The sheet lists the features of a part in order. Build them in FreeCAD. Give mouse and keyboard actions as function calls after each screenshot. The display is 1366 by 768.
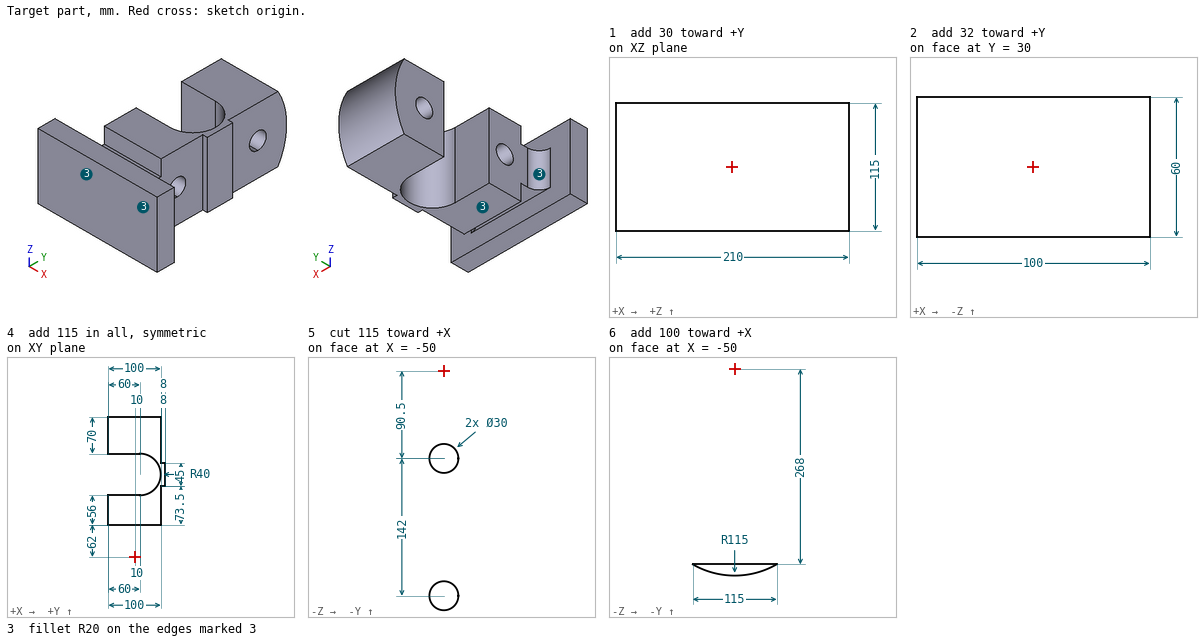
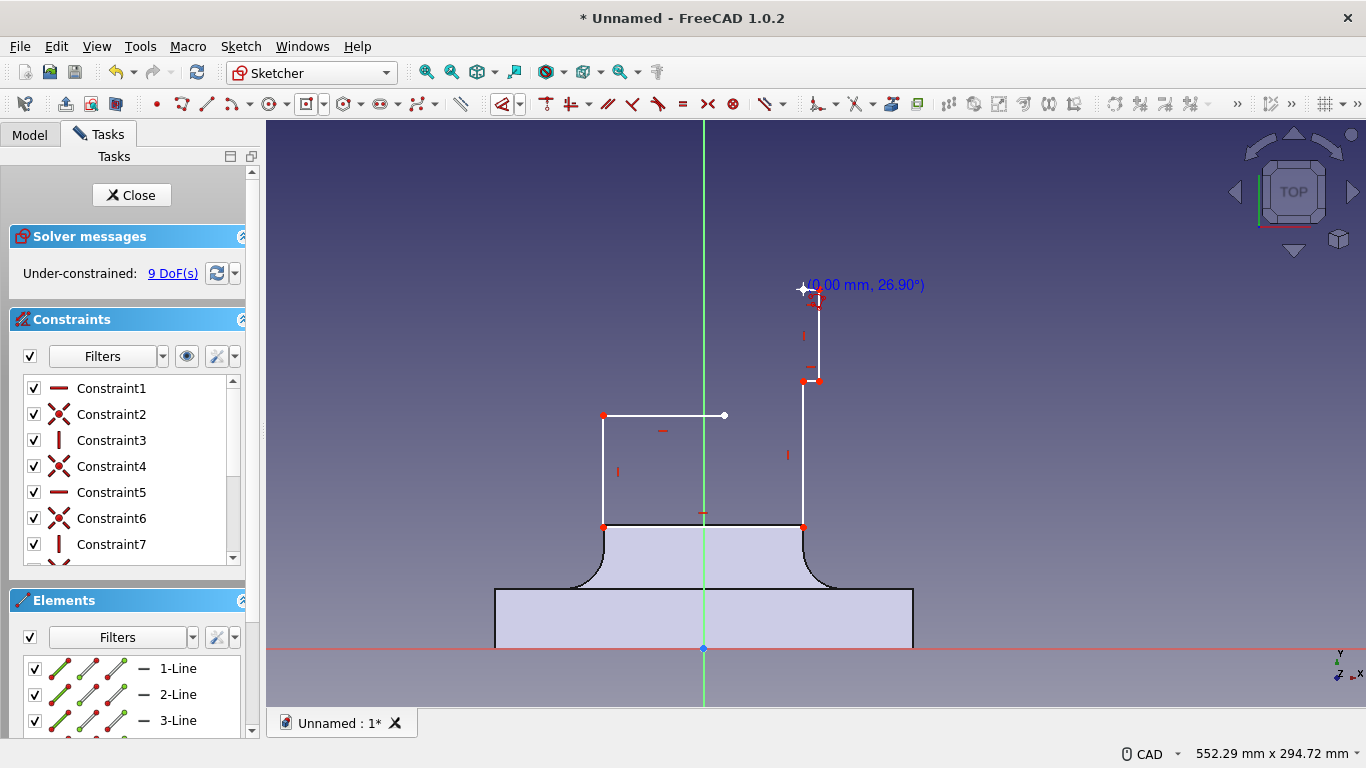
scroll(820, 477, down, 2)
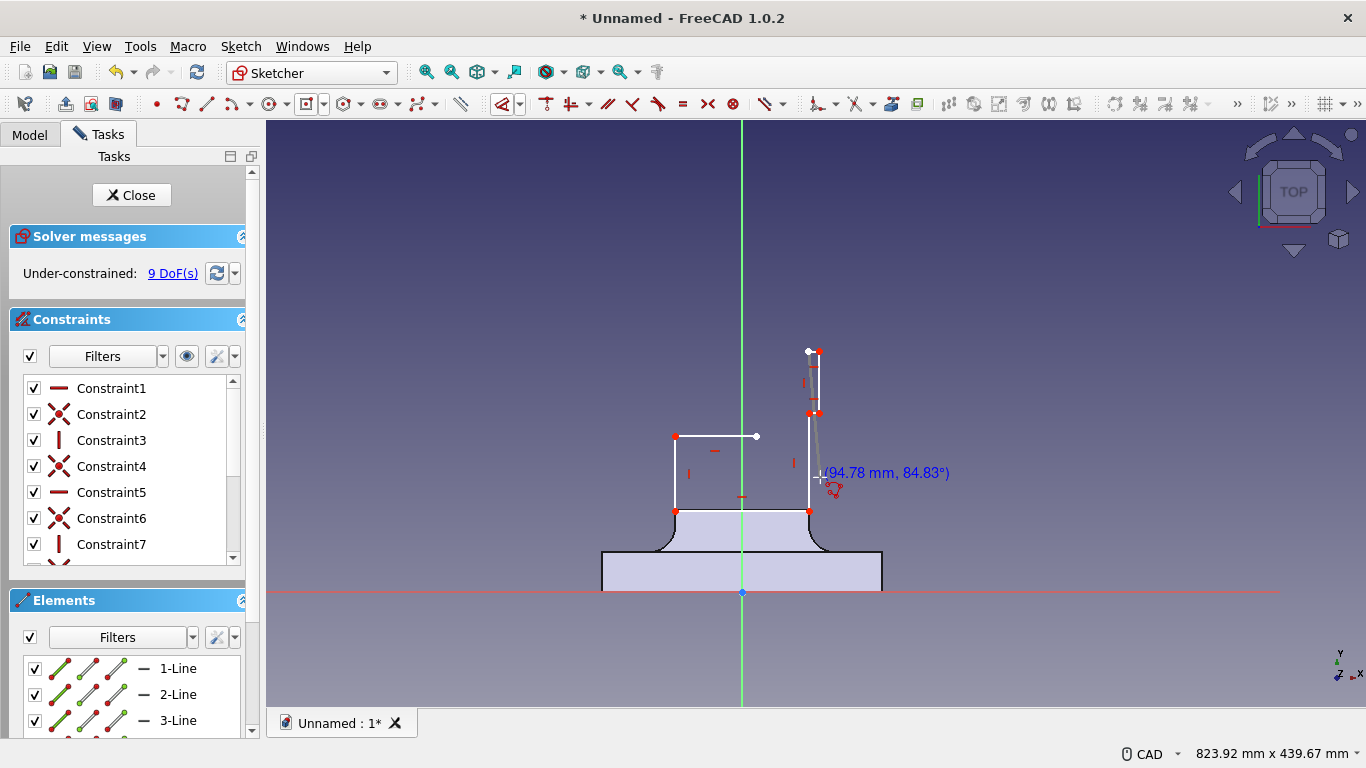
click(809, 235)
click(675, 235)
click(675, 328)
click(756, 328)
right_click(756, 328)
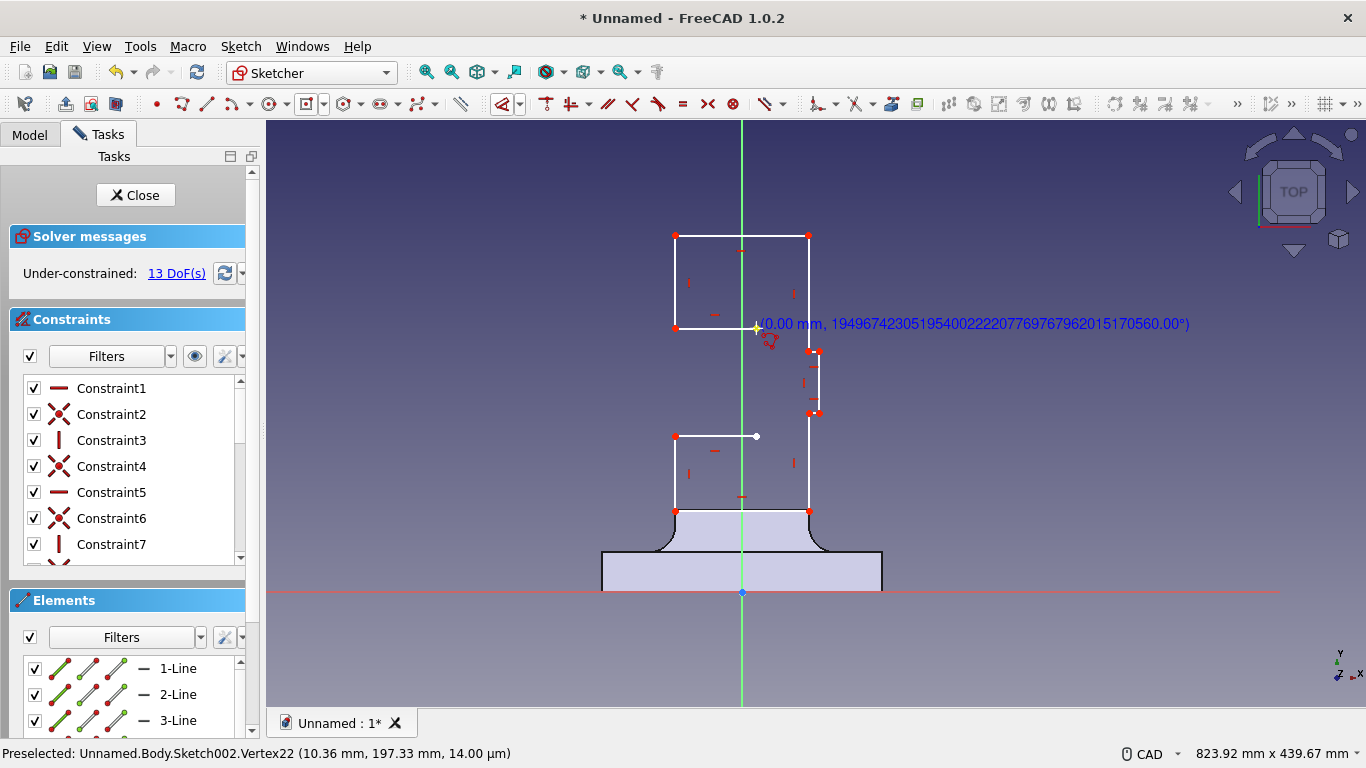
key(g)
key(3)
key(a)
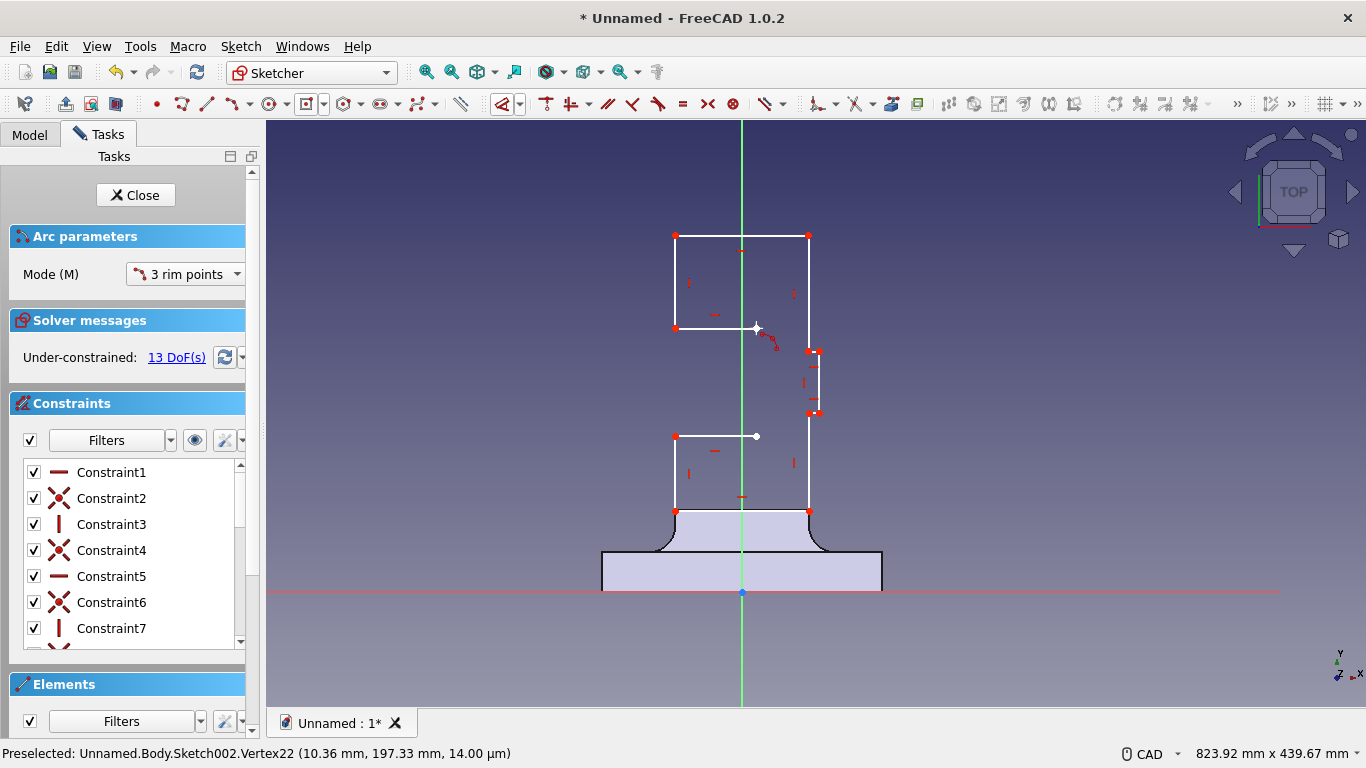
click(756, 329)
click(756, 436)
click(806, 398)
key(Escape)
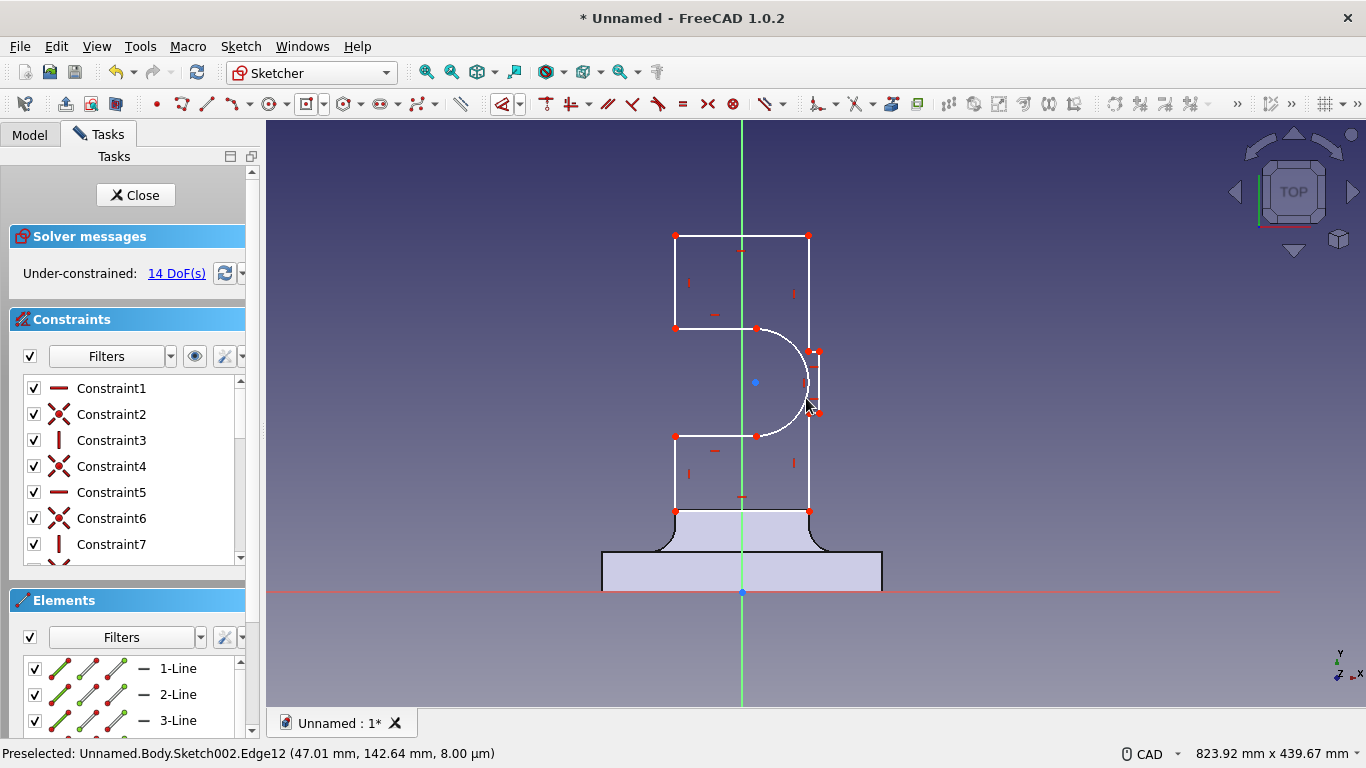
click(502, 104)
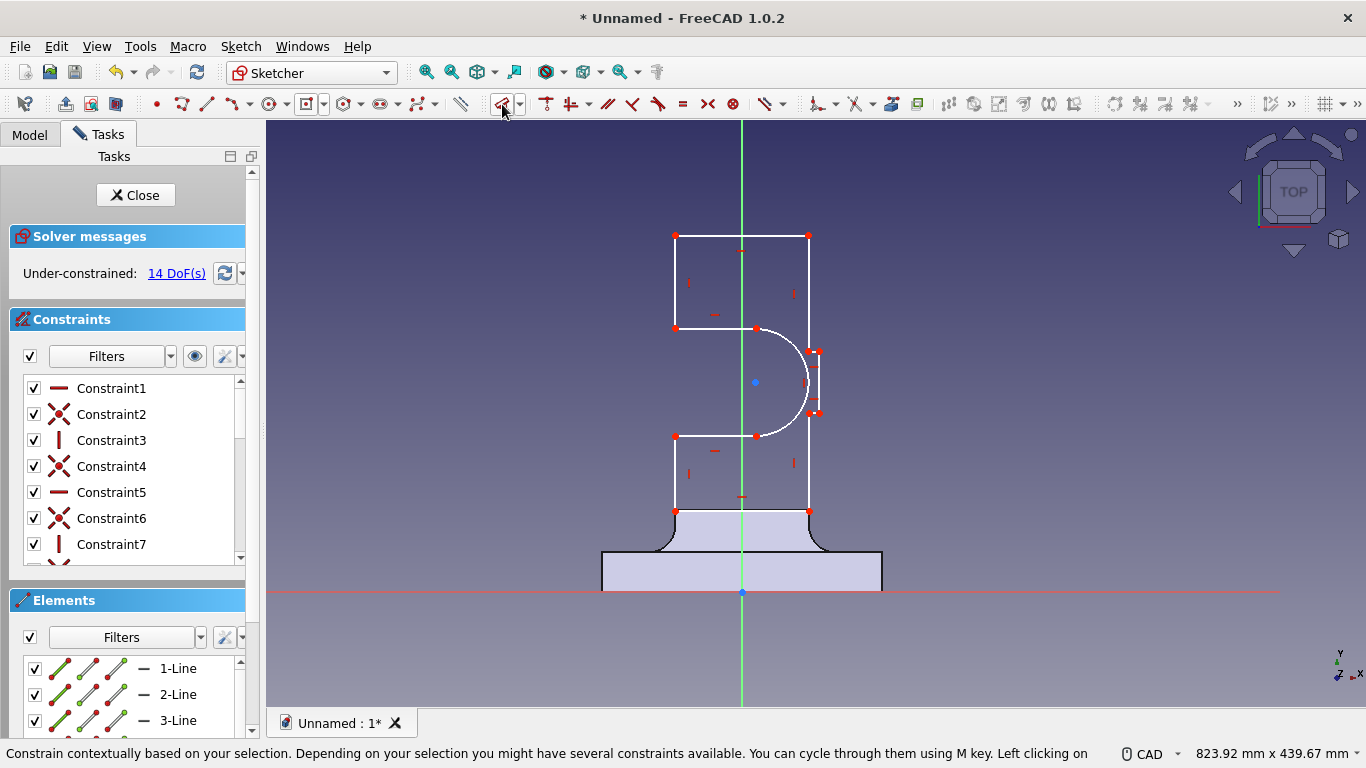
scroll(799, 414, up, 2)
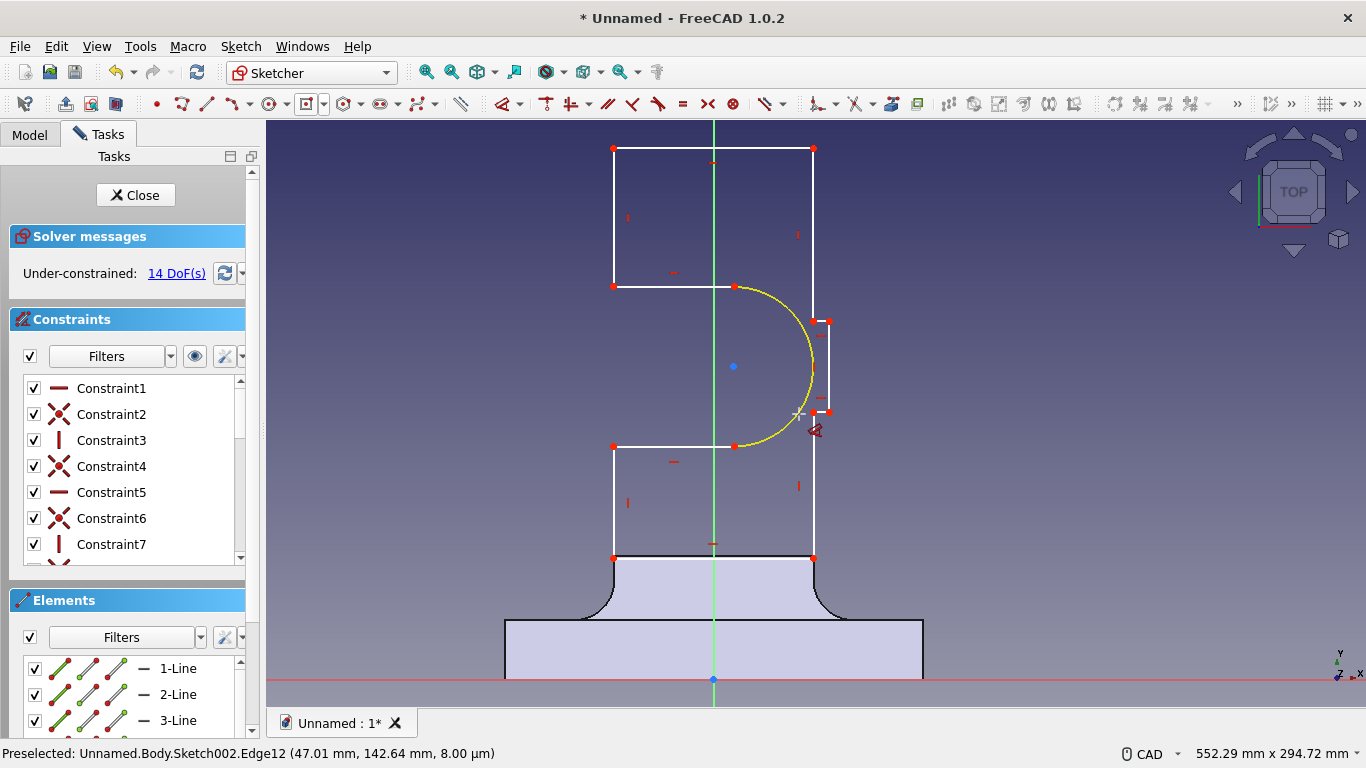
click(798, 413)
click(782, 467)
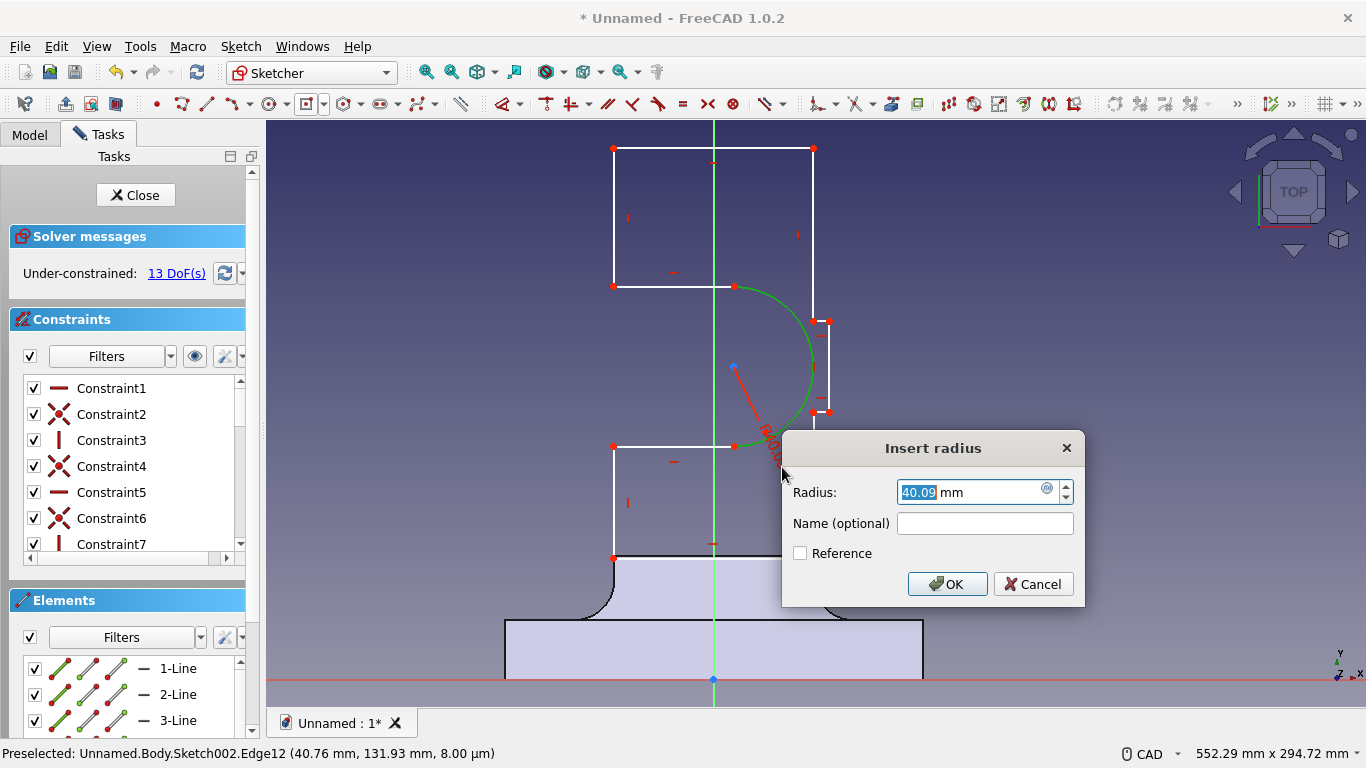
text(40)
key(Return)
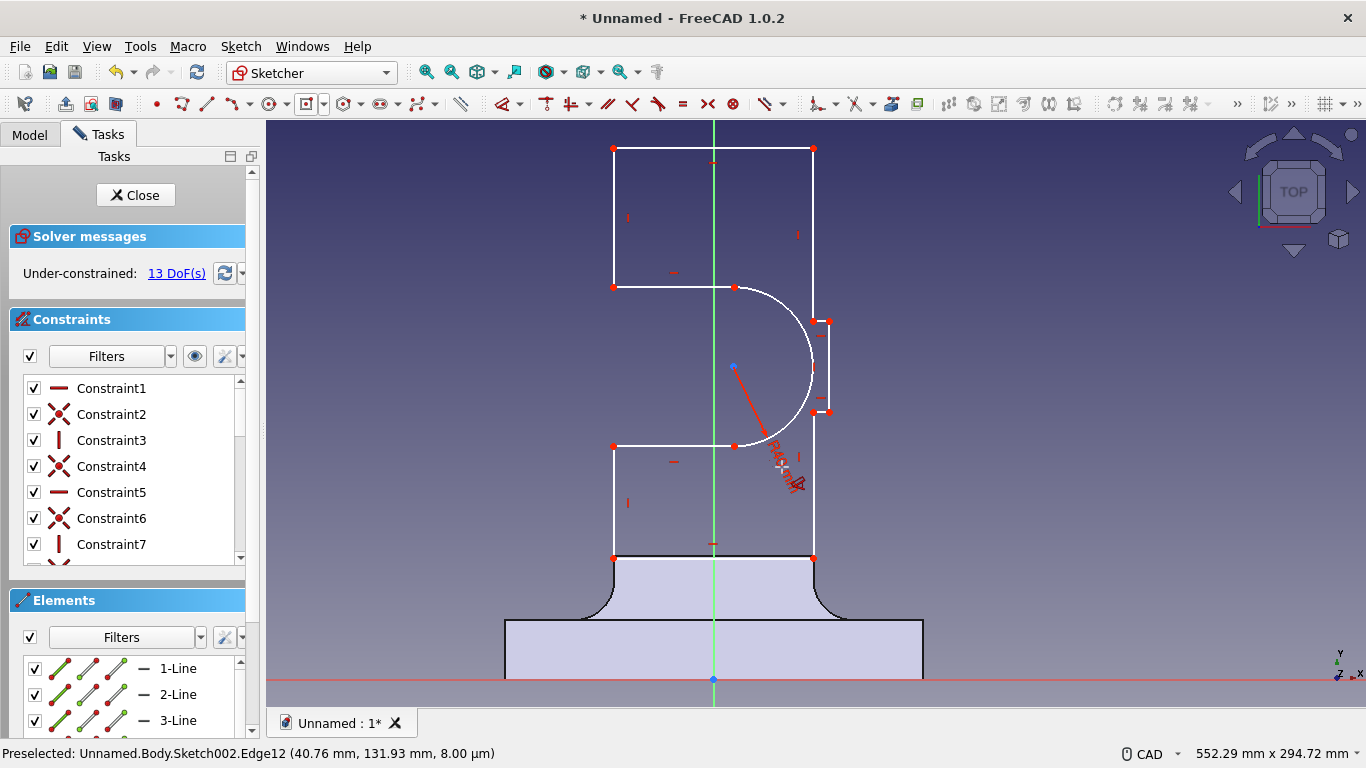
scroll(822, 412, up, 5)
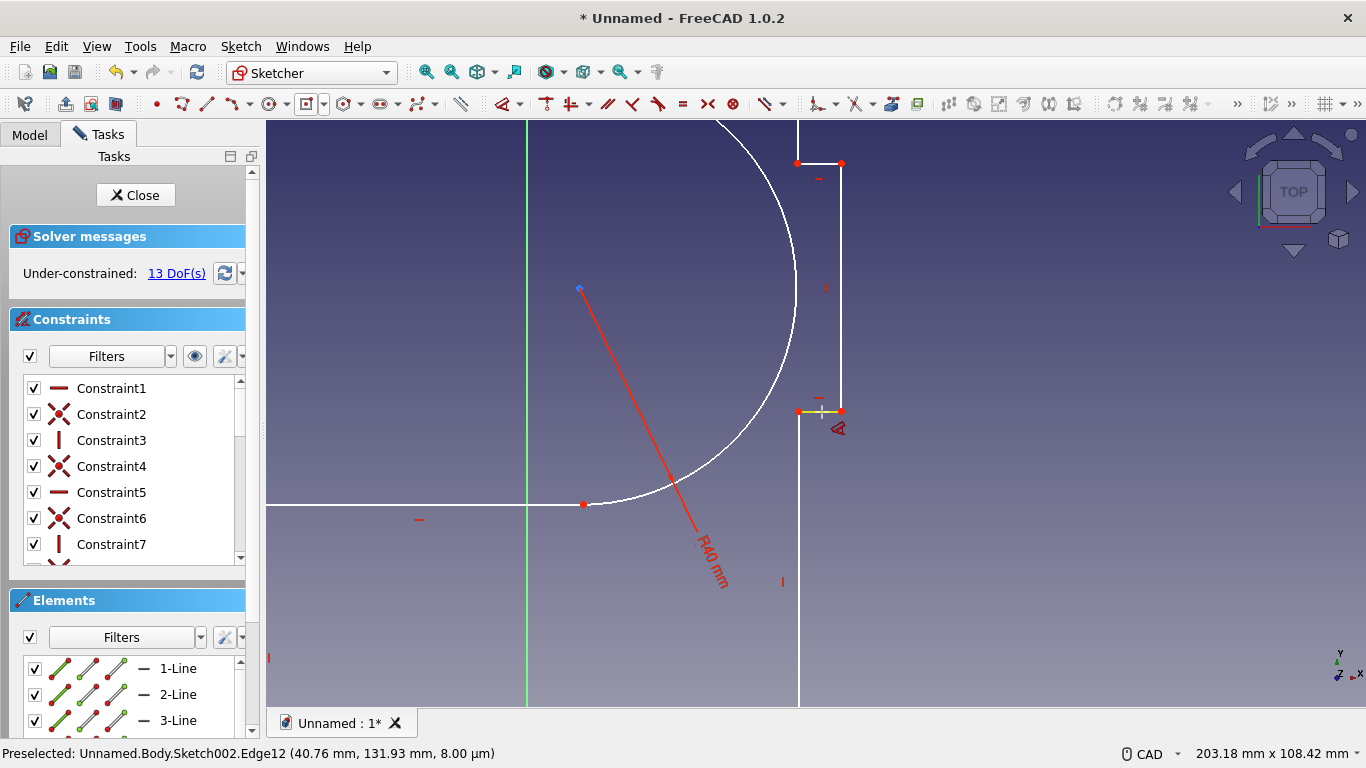
click(820, 412)
click(820, 378)